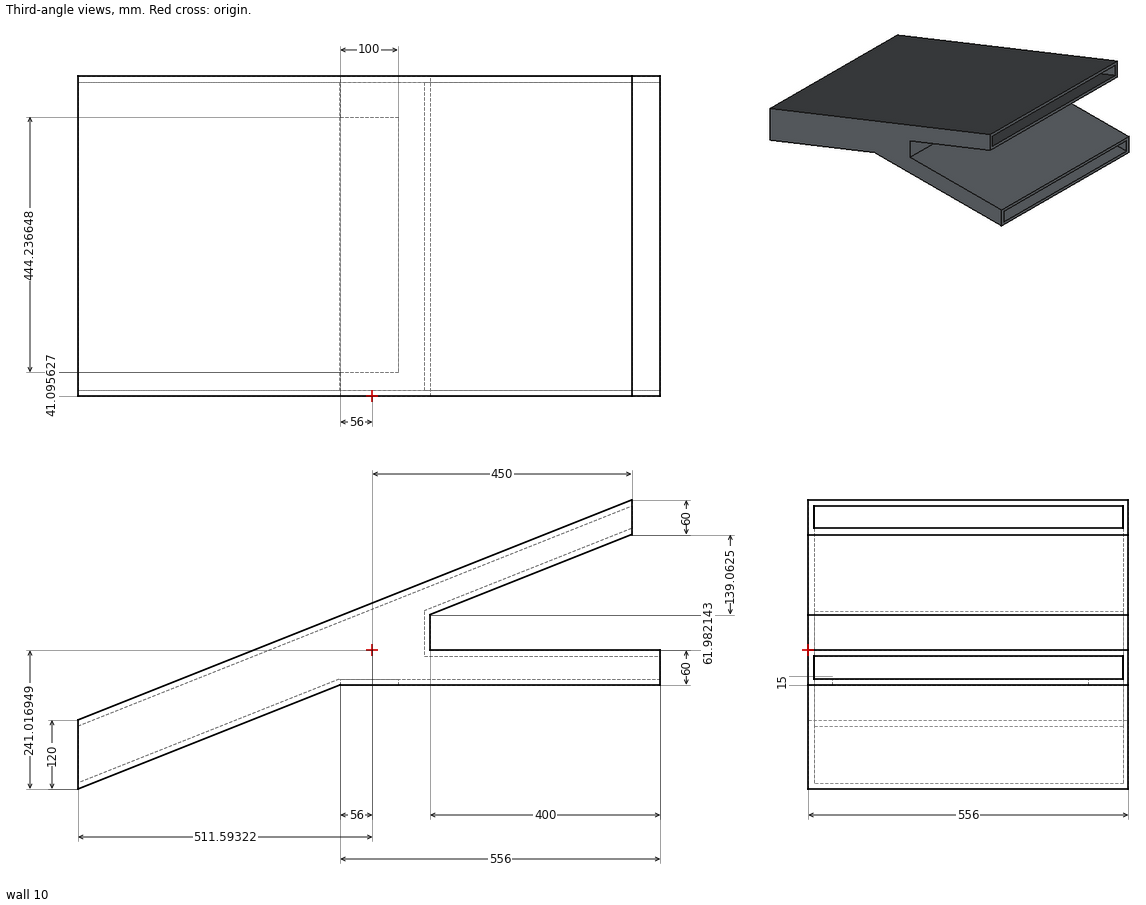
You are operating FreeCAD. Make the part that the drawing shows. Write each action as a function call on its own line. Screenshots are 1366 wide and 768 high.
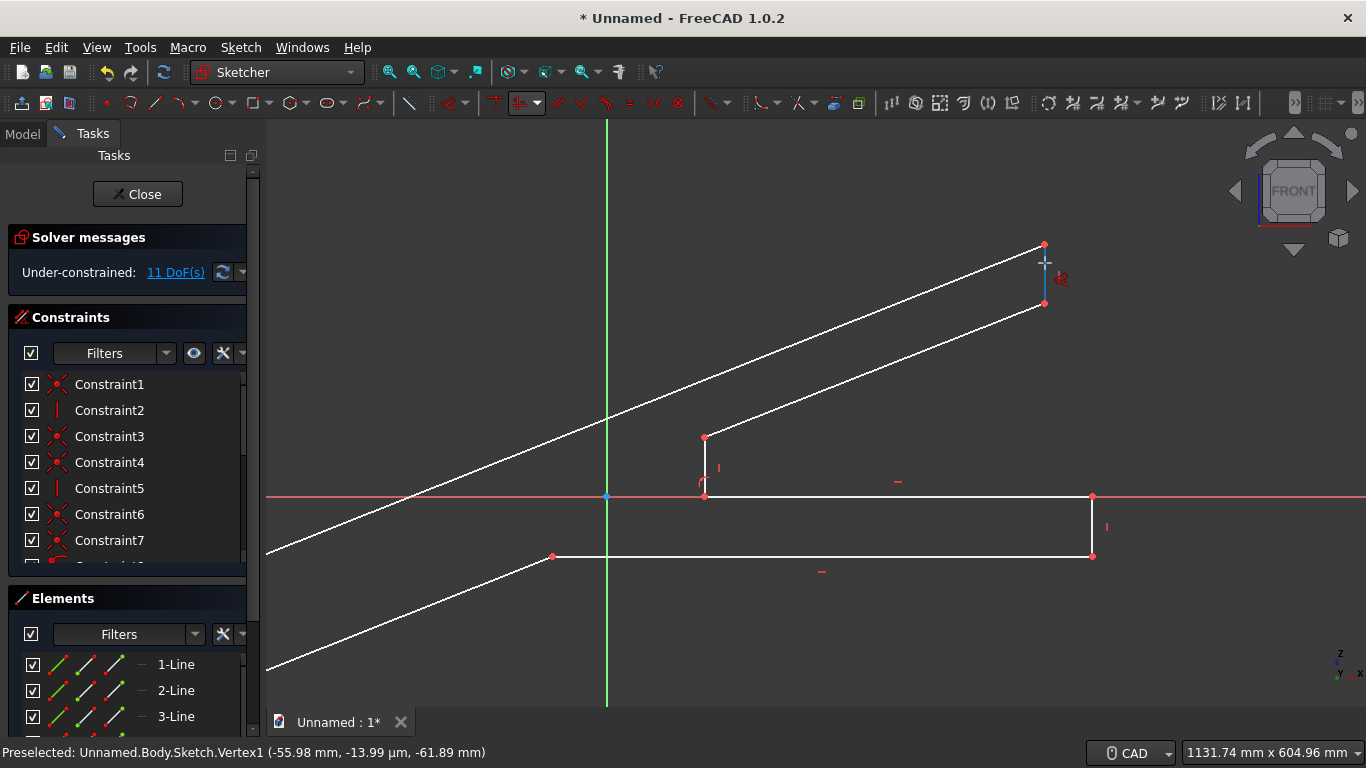
click(1045, 262)
click(1079, 274)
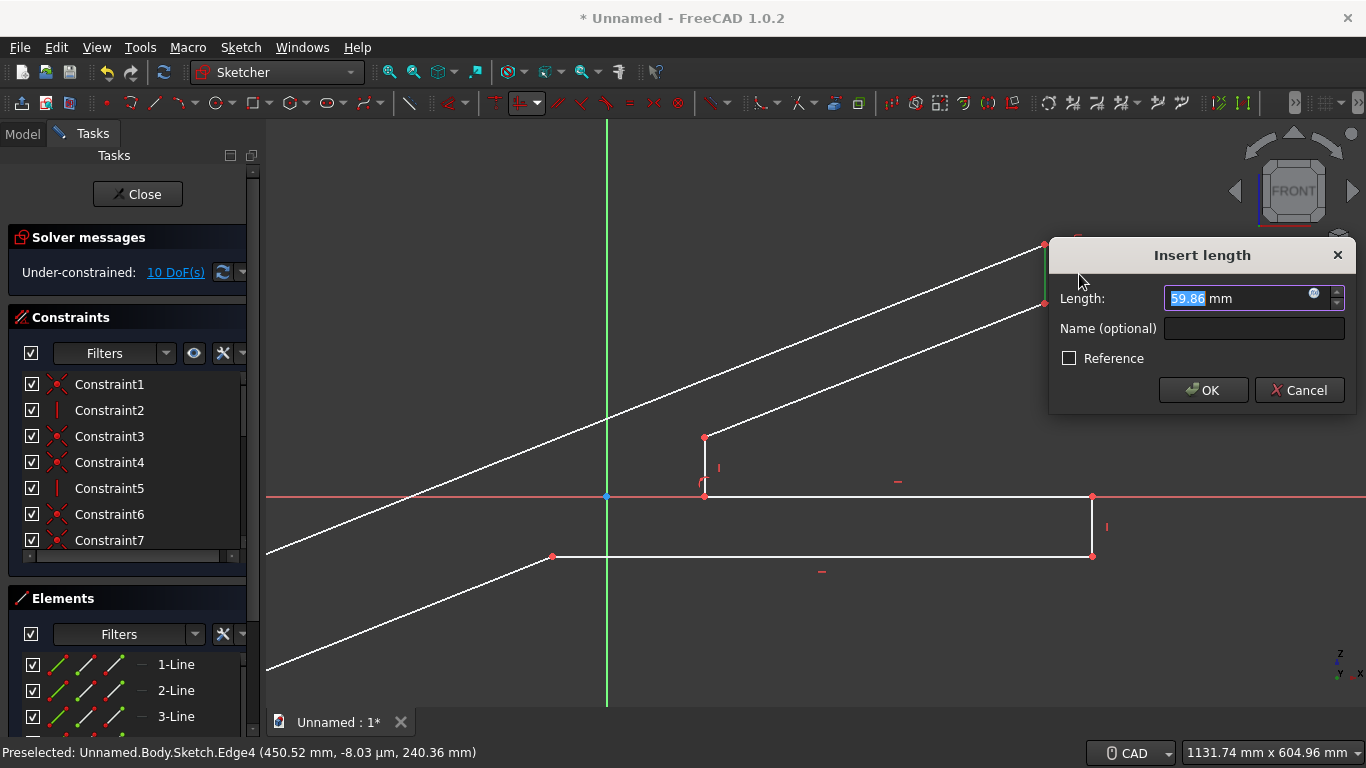
text(60)
key(Return)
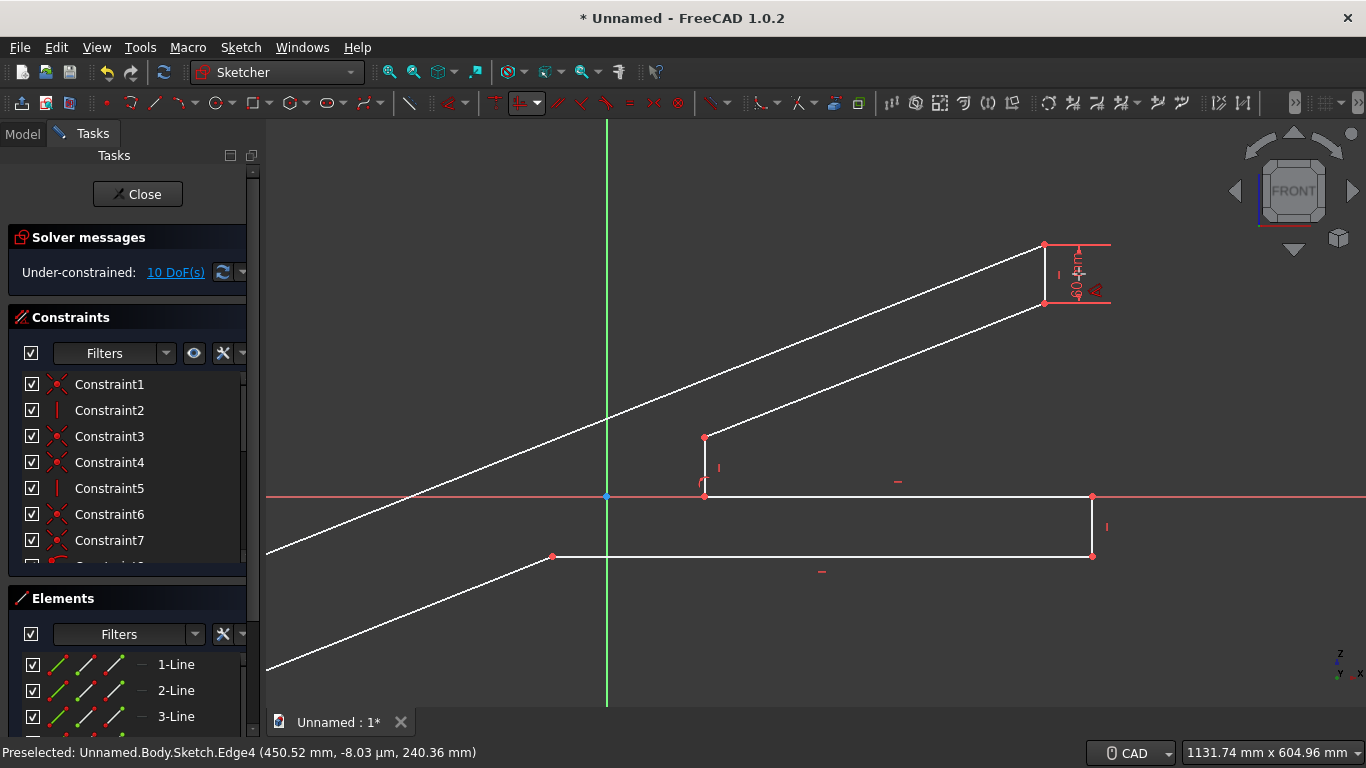
click(1092, 515)
click(1126, 527)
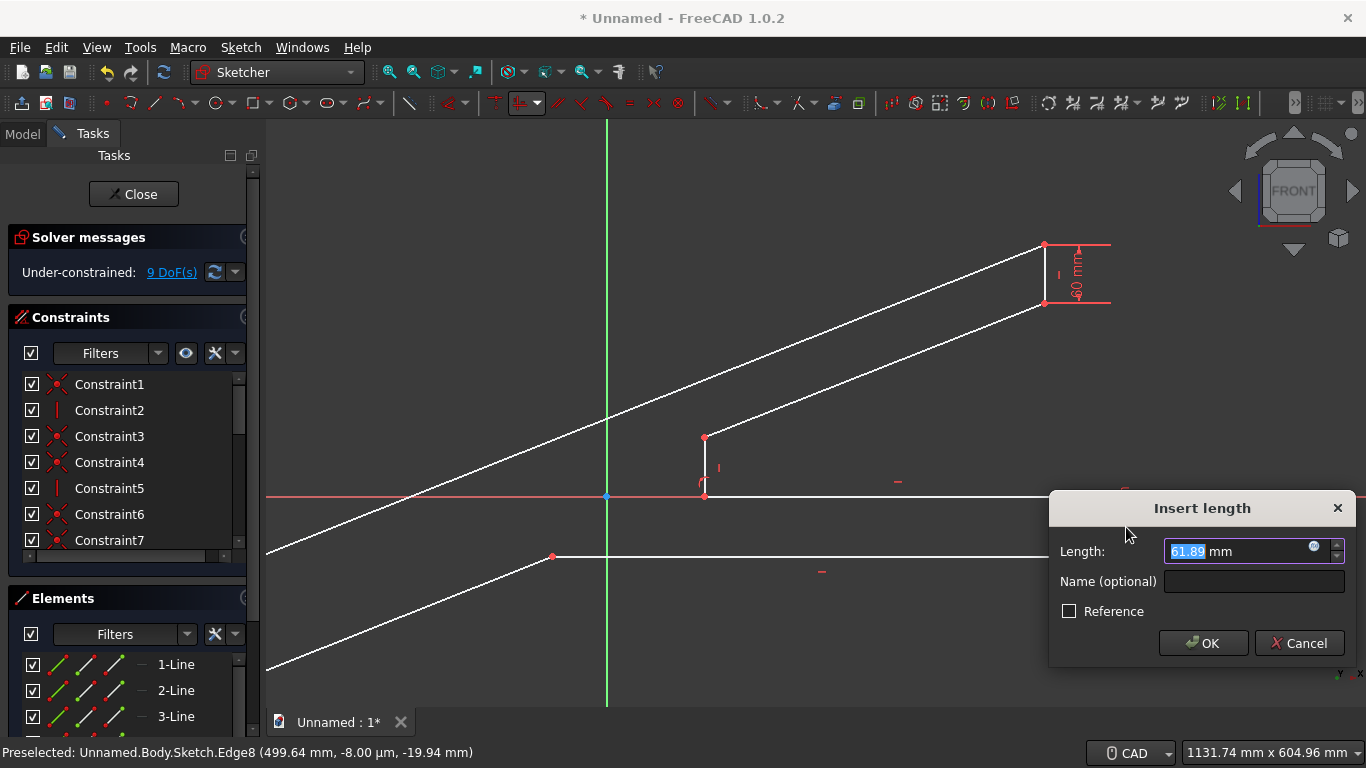
text(60)
key(Return)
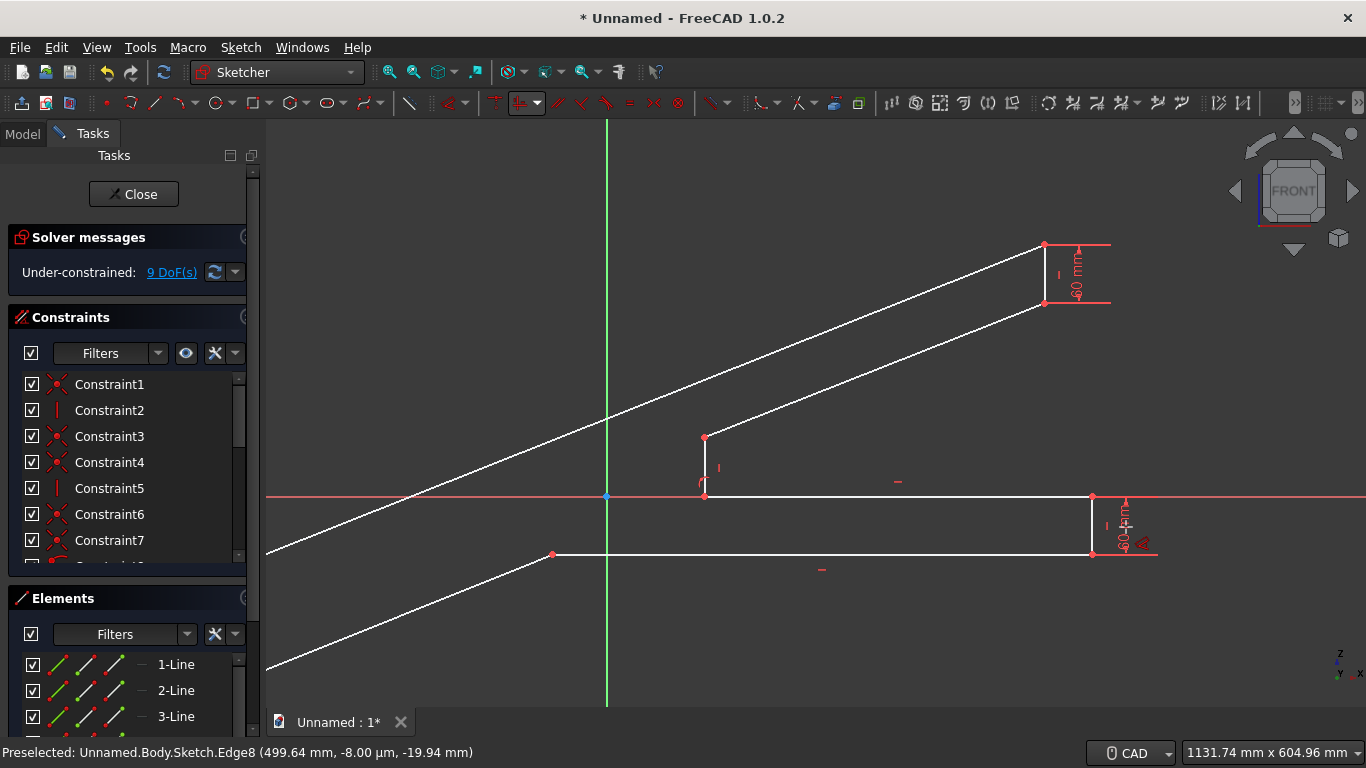
scroll(1045, 263, down, 2)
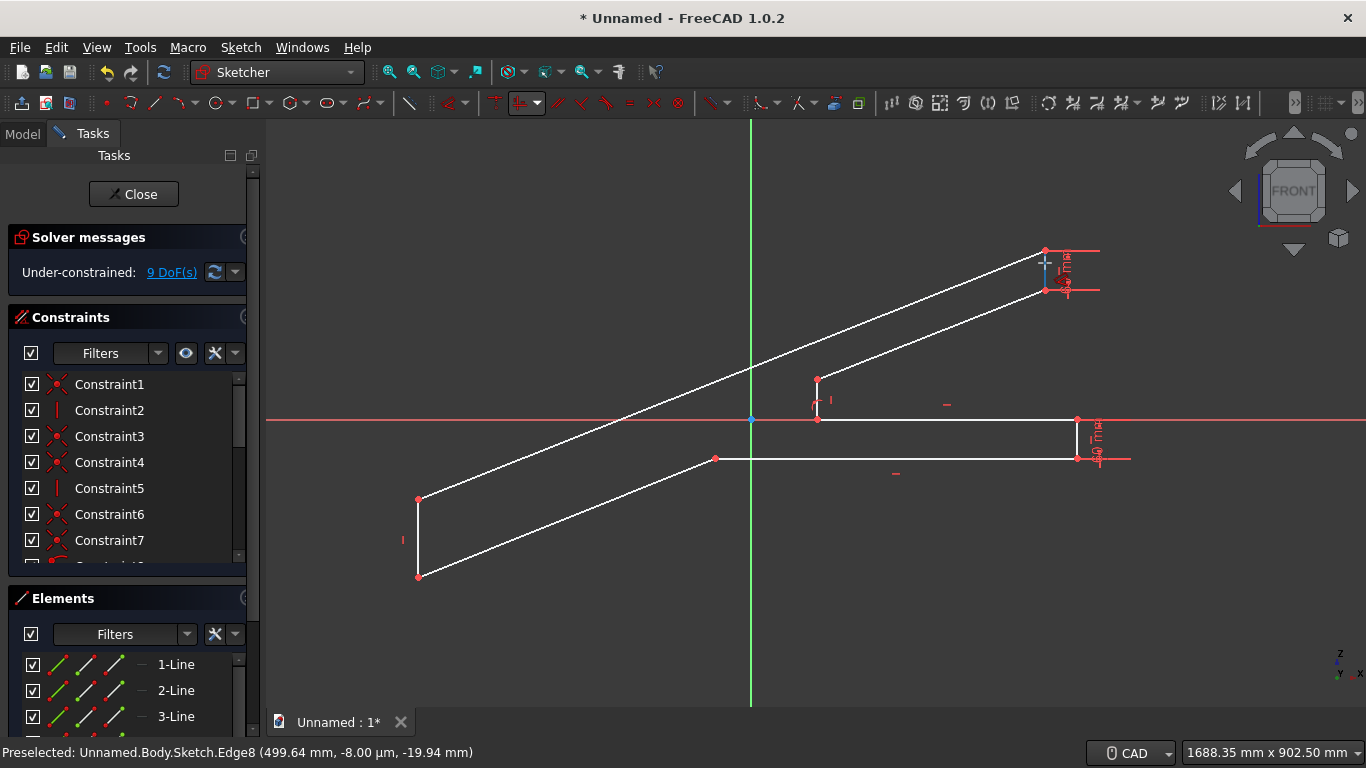
click(418, 555)
click(384, 539)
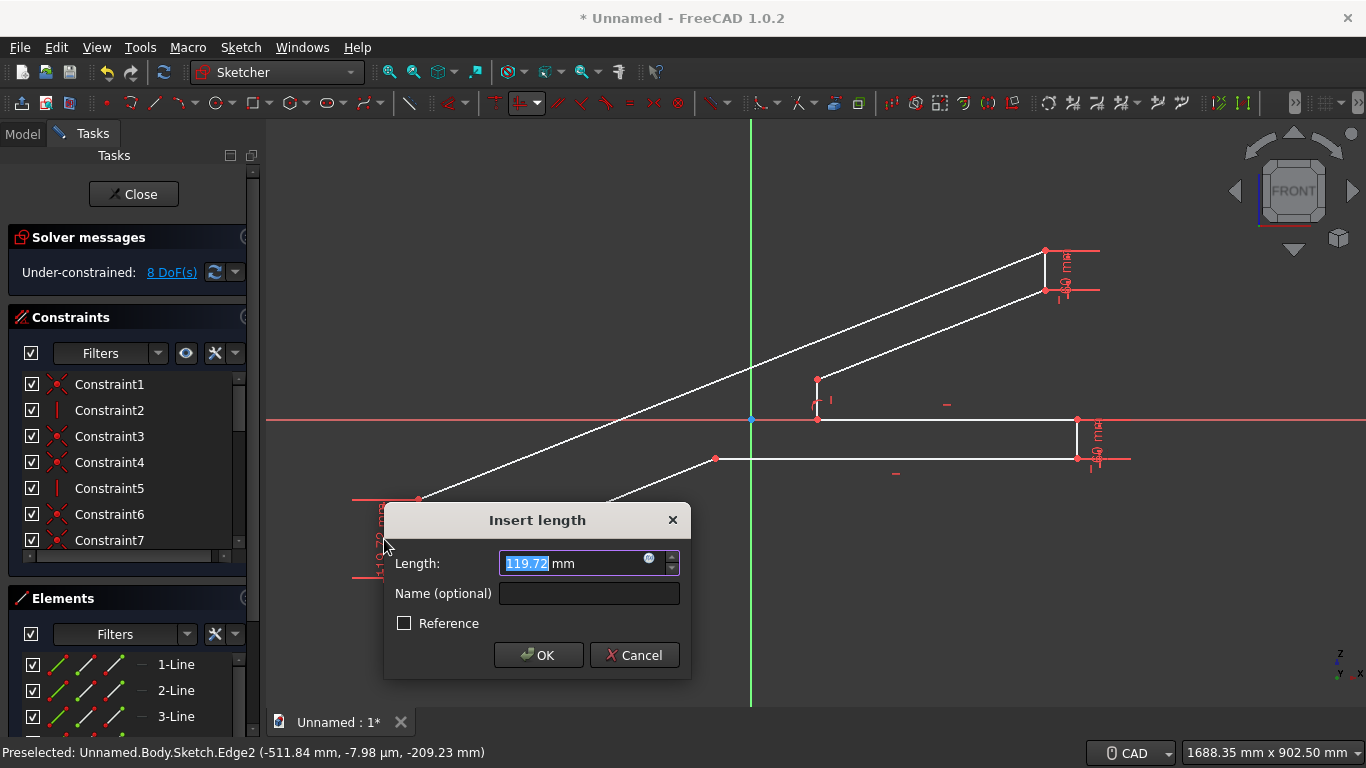
text(120)
key(Return)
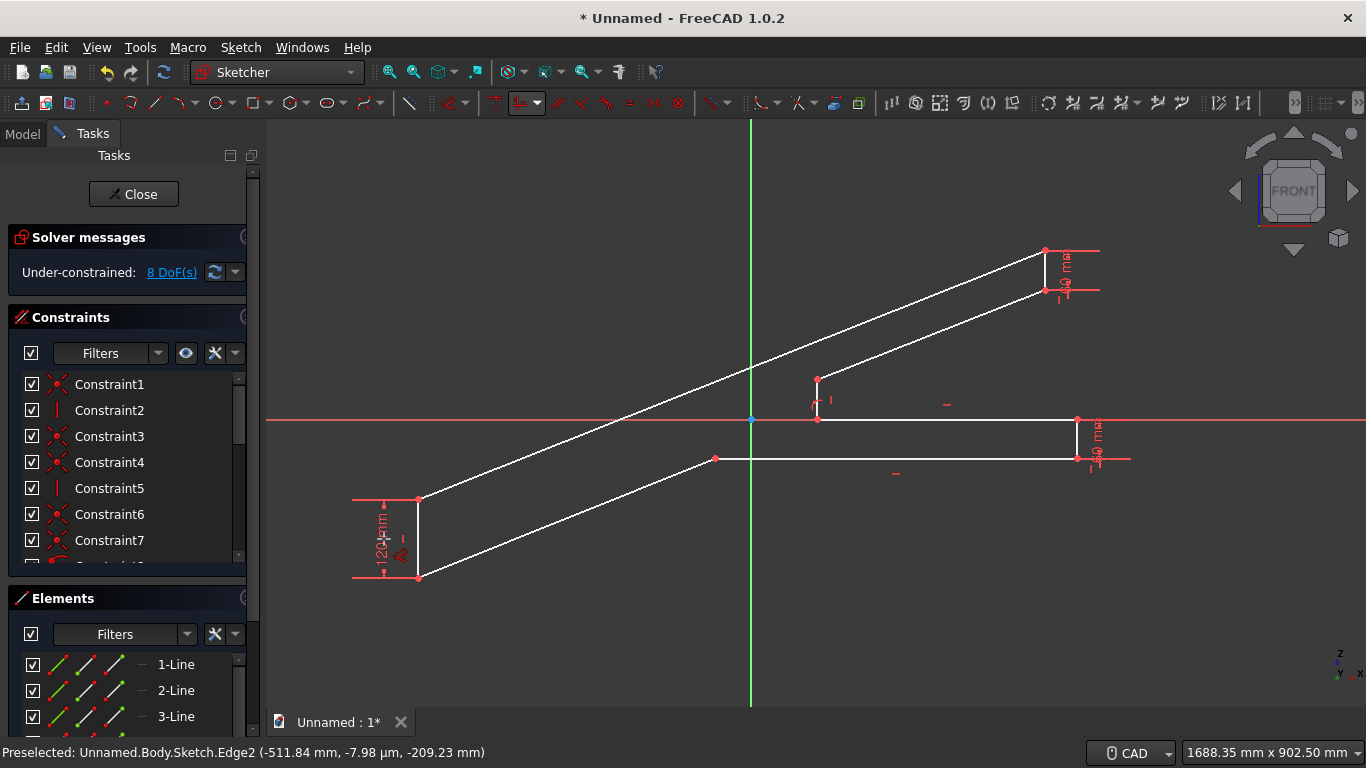
click(895, 420)
click(947, 386)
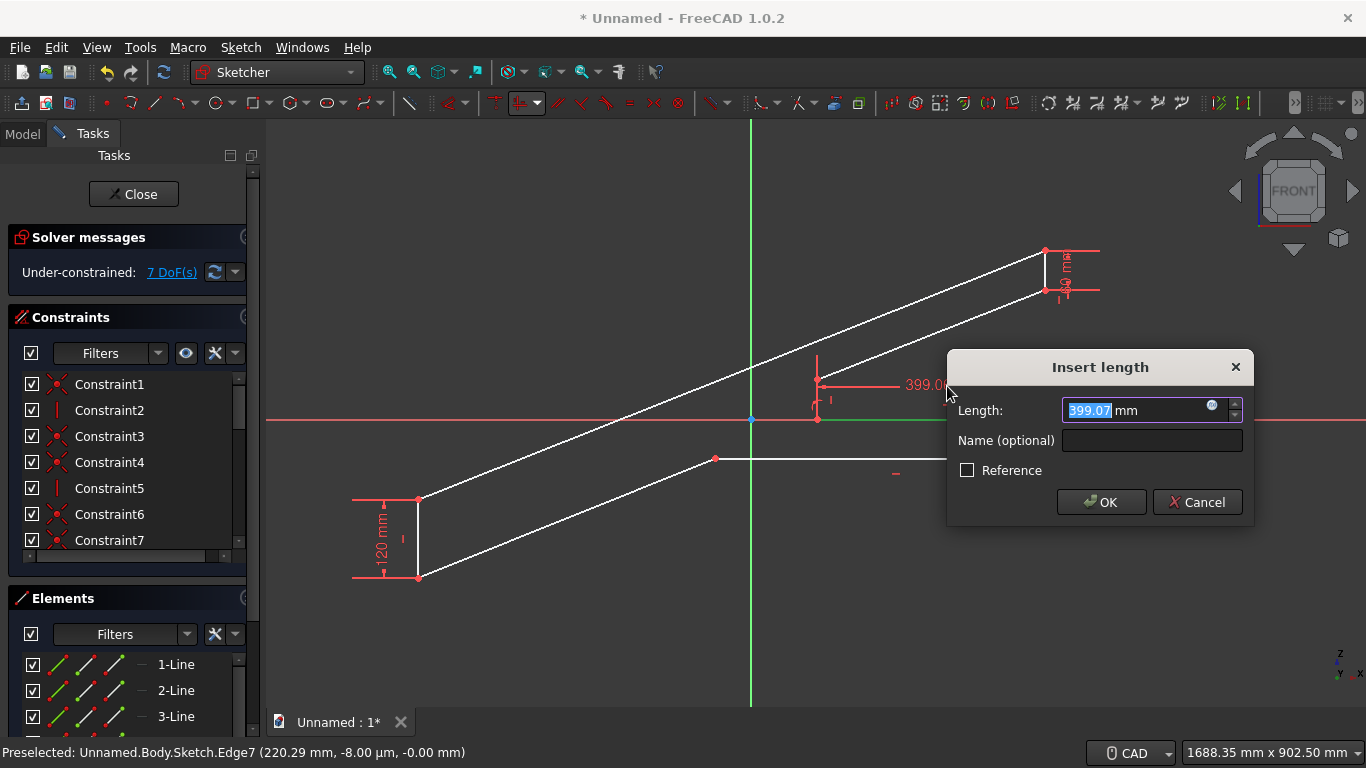
text(400)
key(Return)